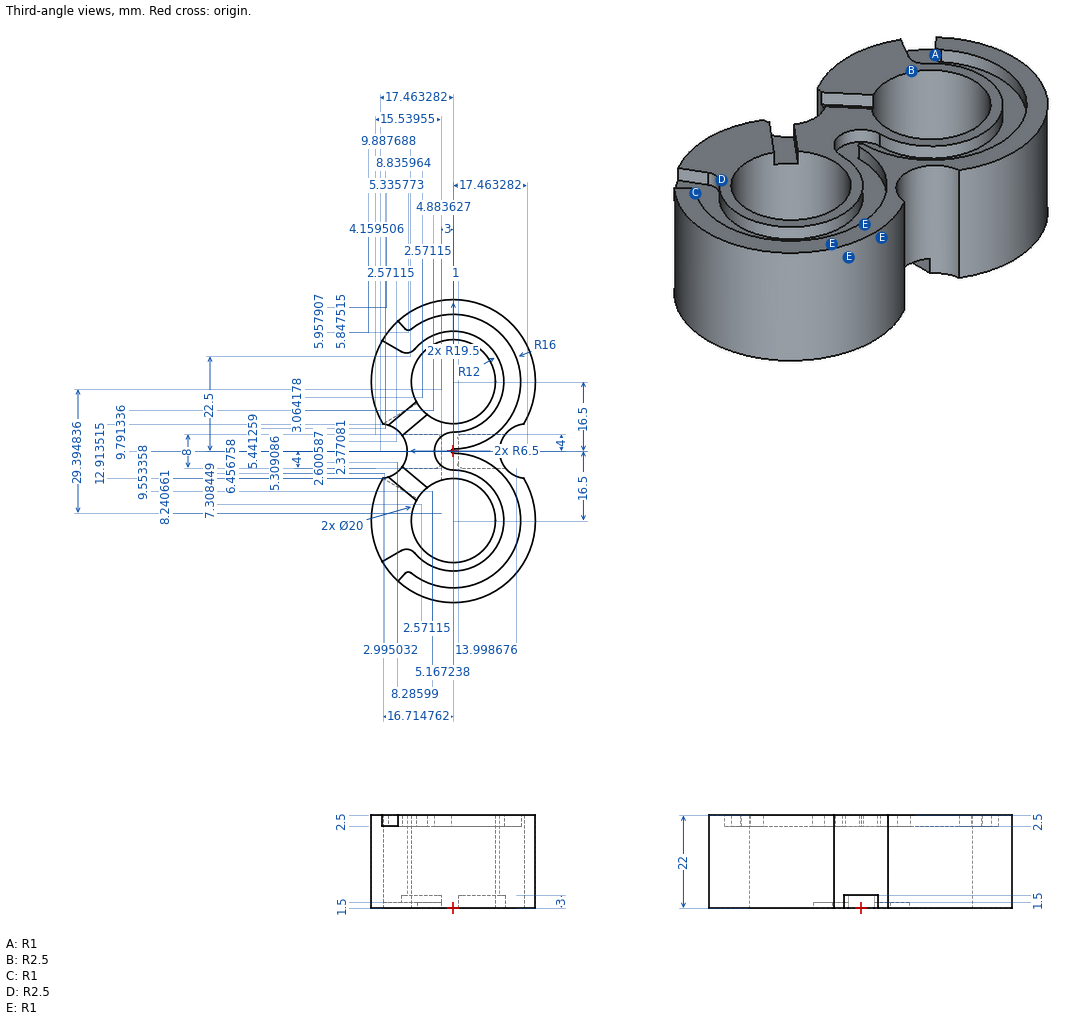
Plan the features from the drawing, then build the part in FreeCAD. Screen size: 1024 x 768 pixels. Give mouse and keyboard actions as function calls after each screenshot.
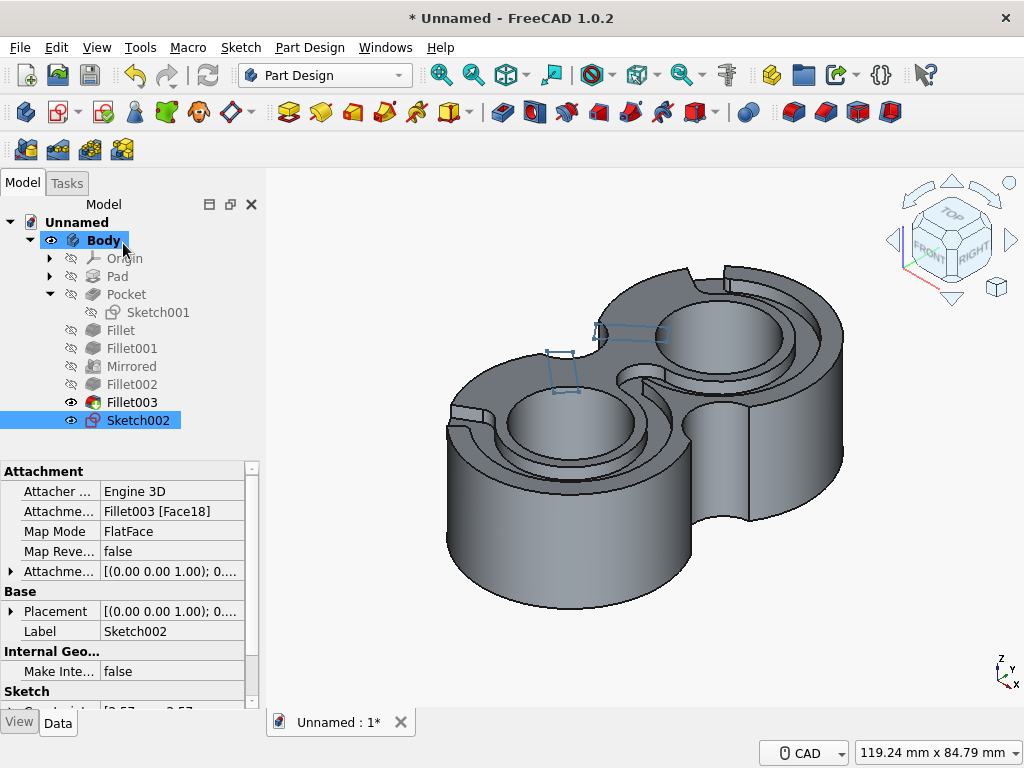
click(504, 112)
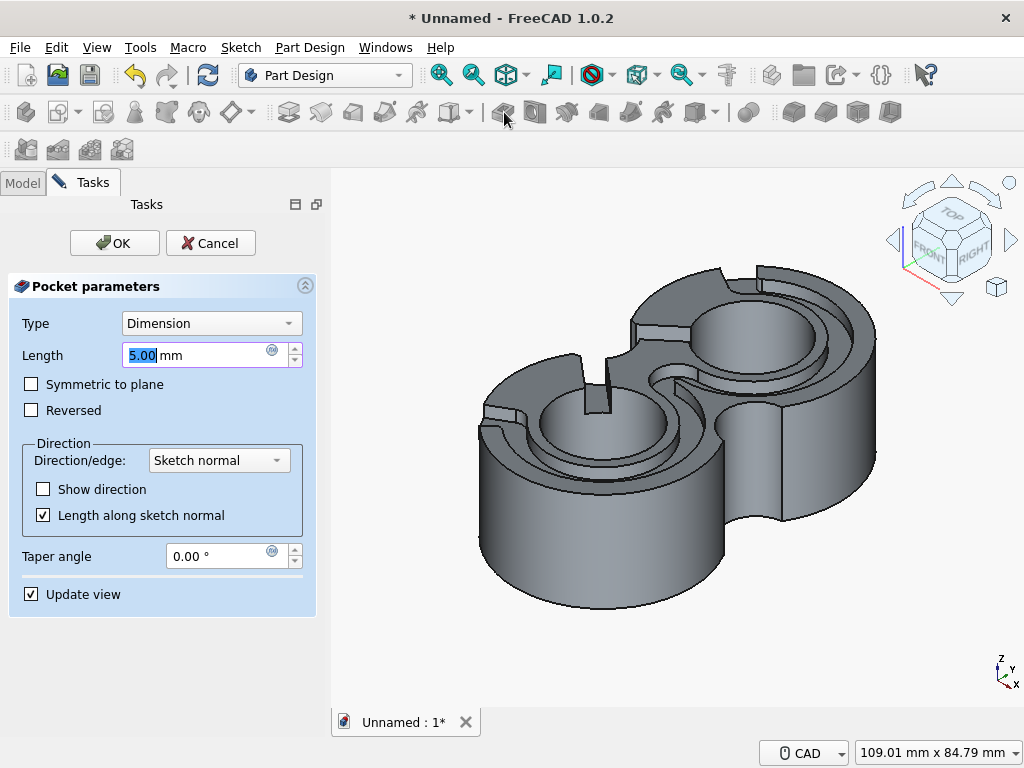
text(2.5)
key(Tab)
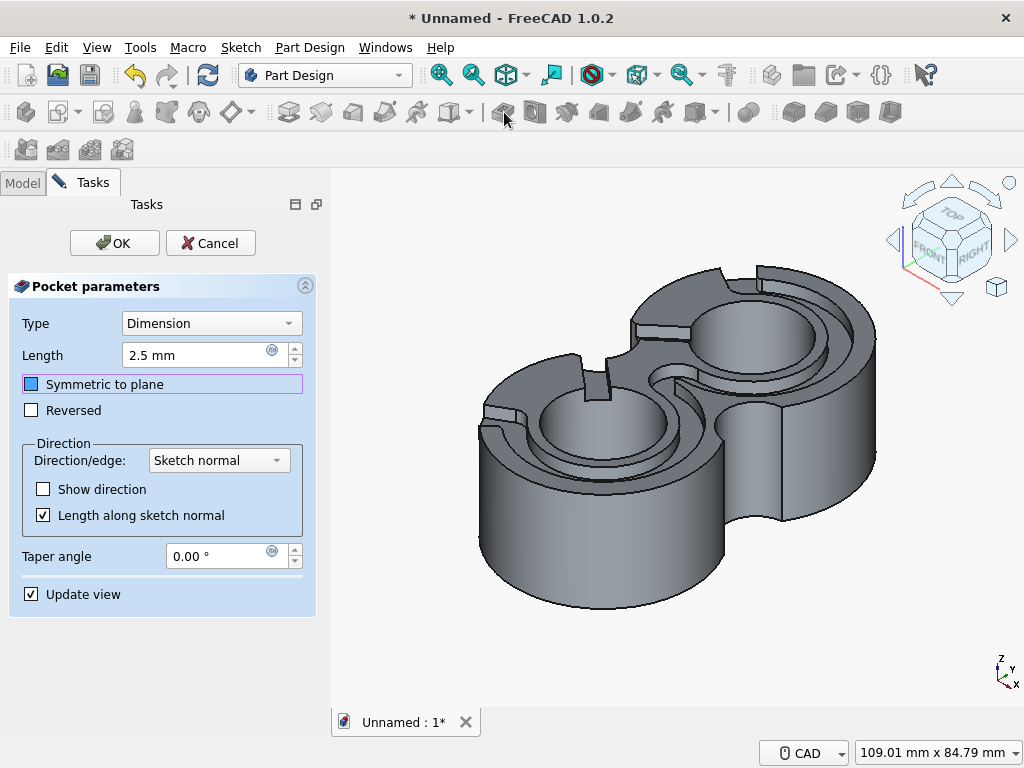
click(115, 243)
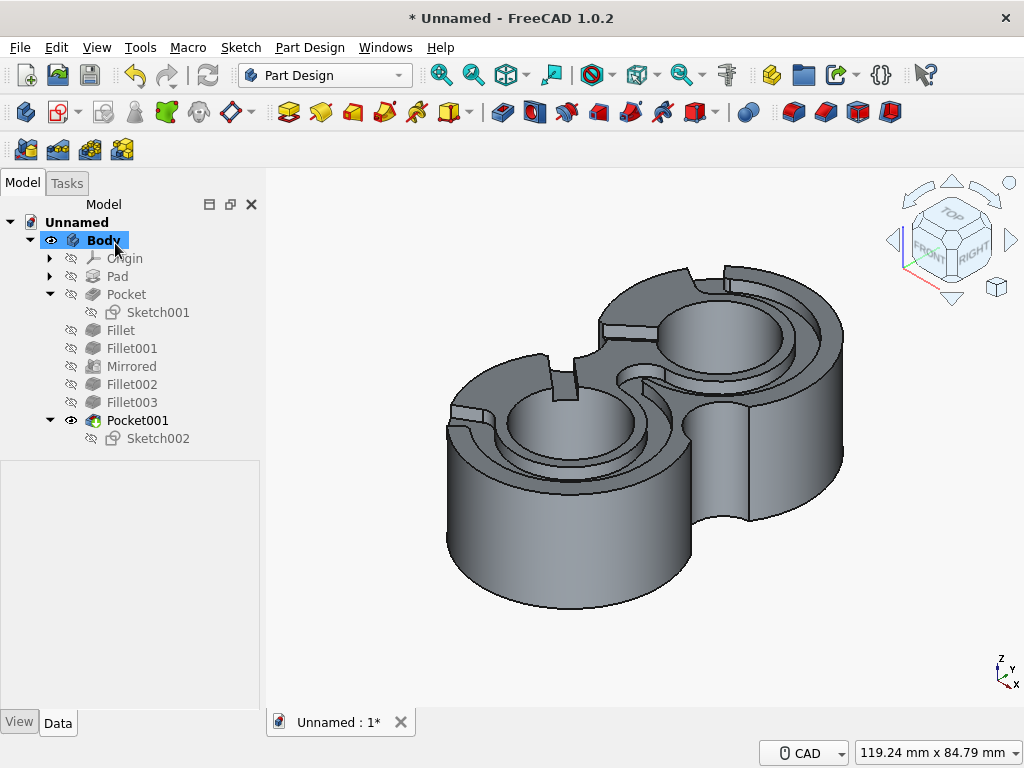
click(58, 112)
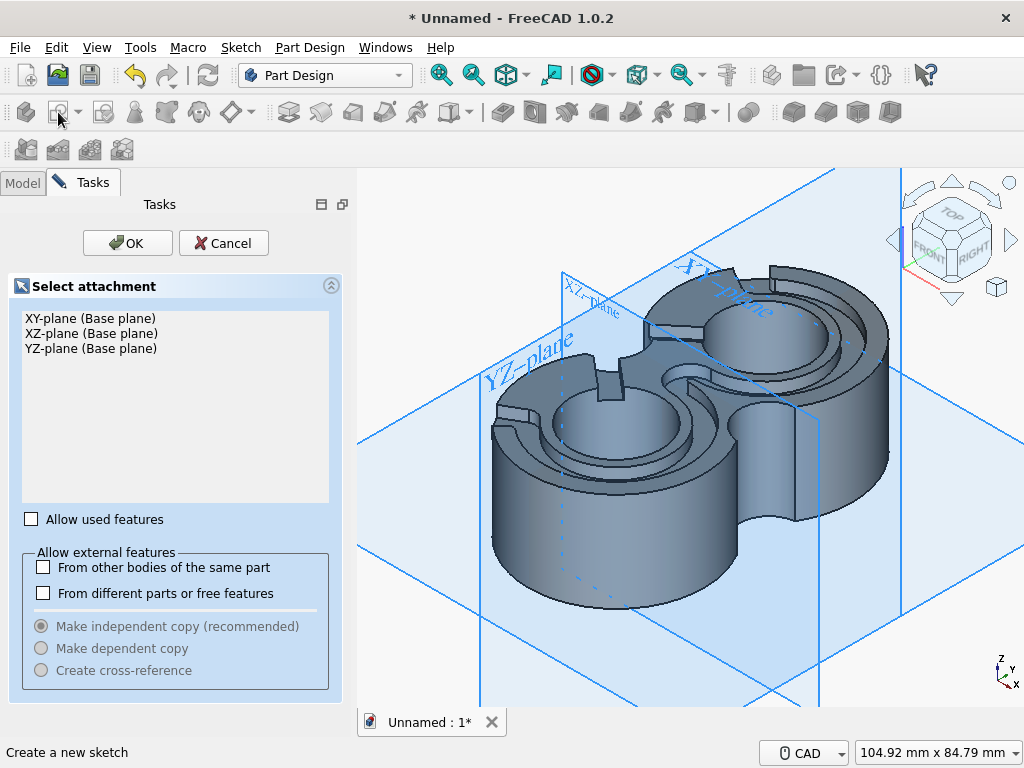
click(82, 318)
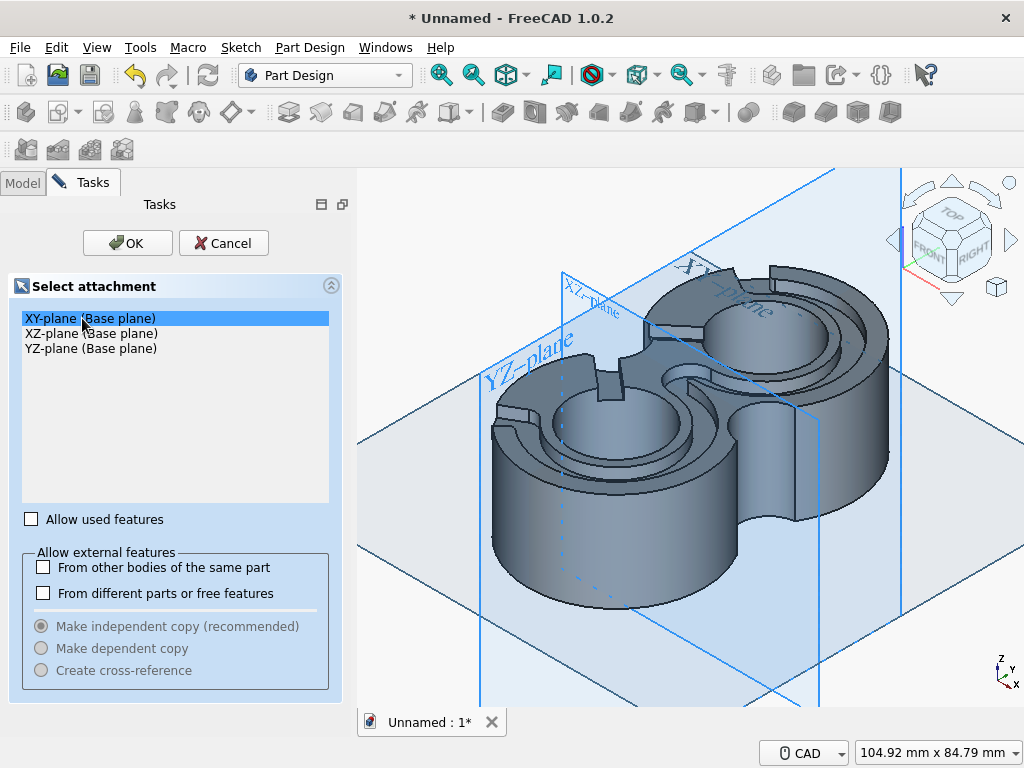
click(128, 243)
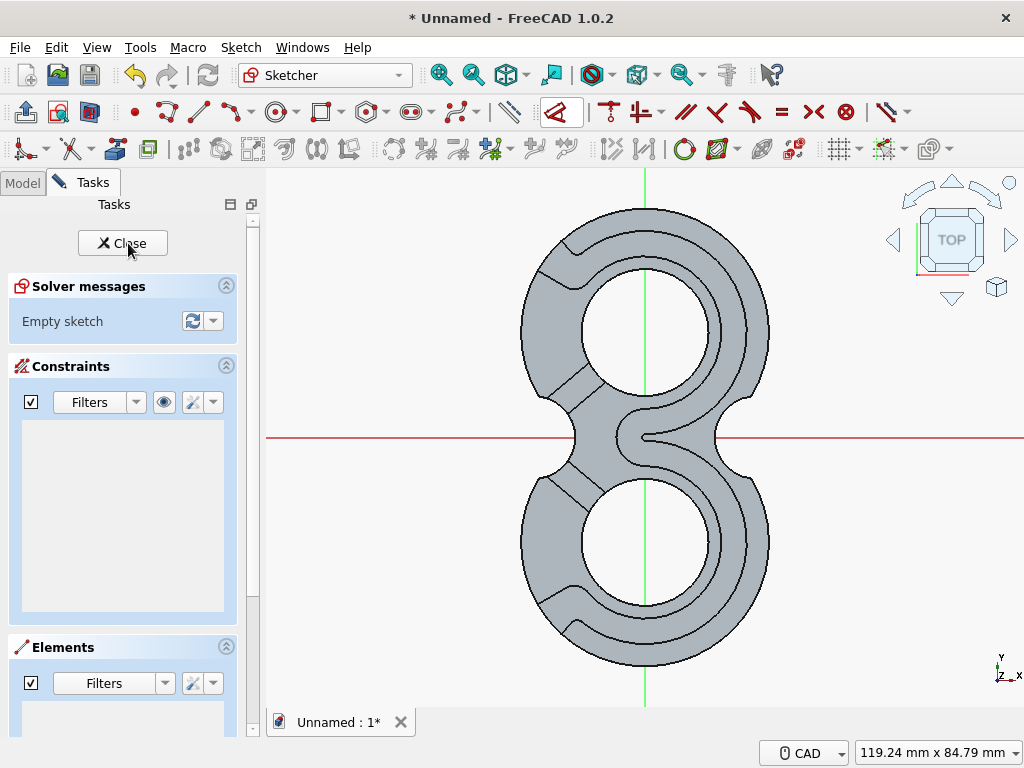
key(q)
key(s)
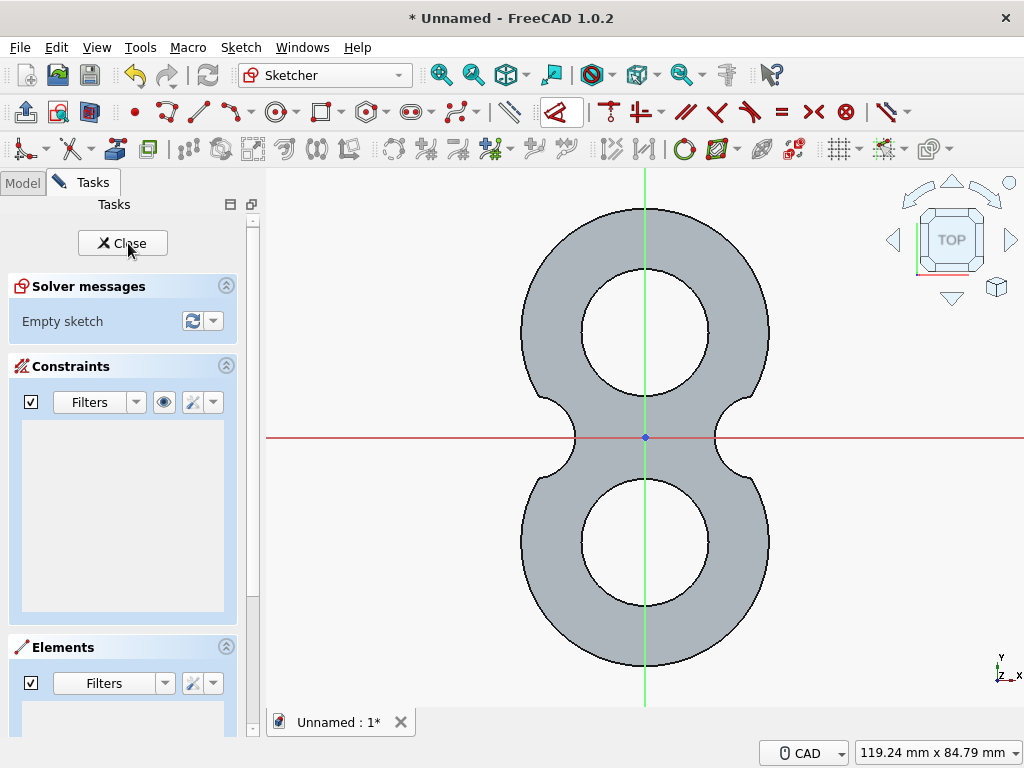
scroll(611, 437, up, 3)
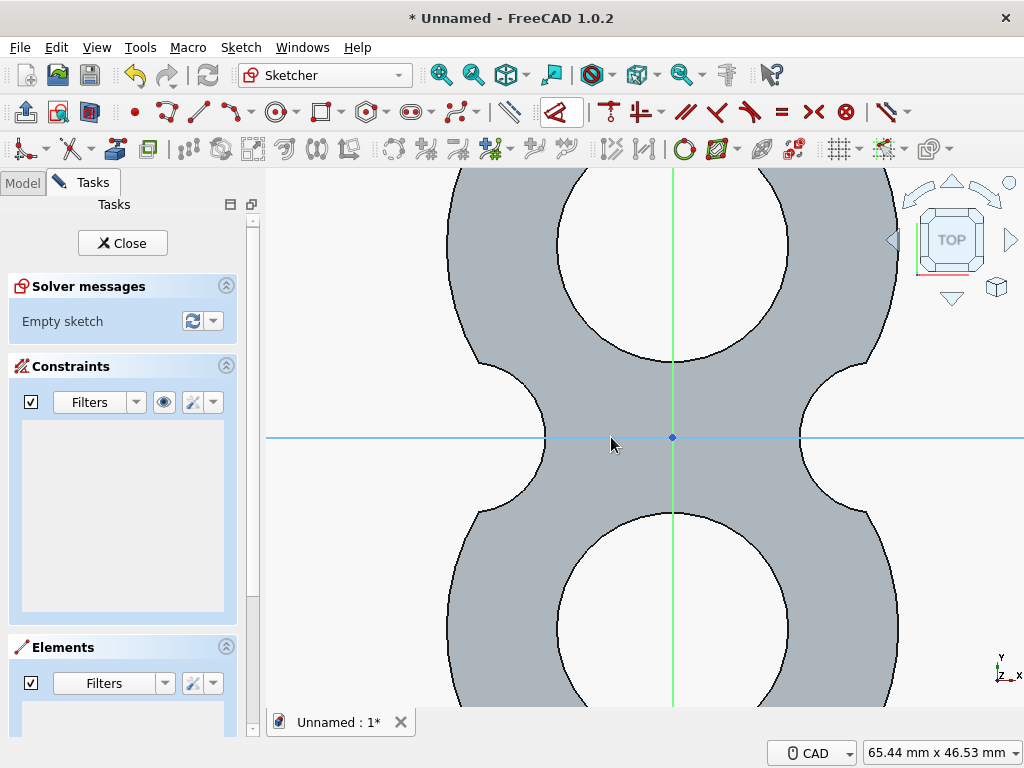
click(168, 112)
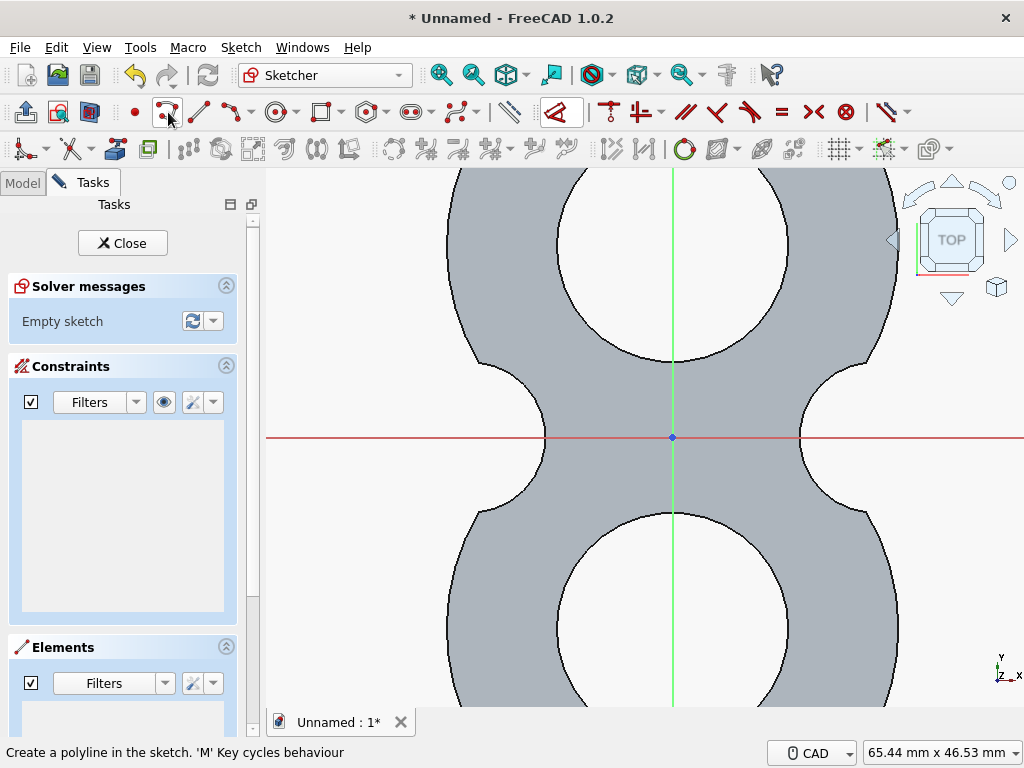
click(638, 267)
click(638, 608)
click(479, 512)
click(479, 363)
click(638, 268)
key(Escape)
key(Escape)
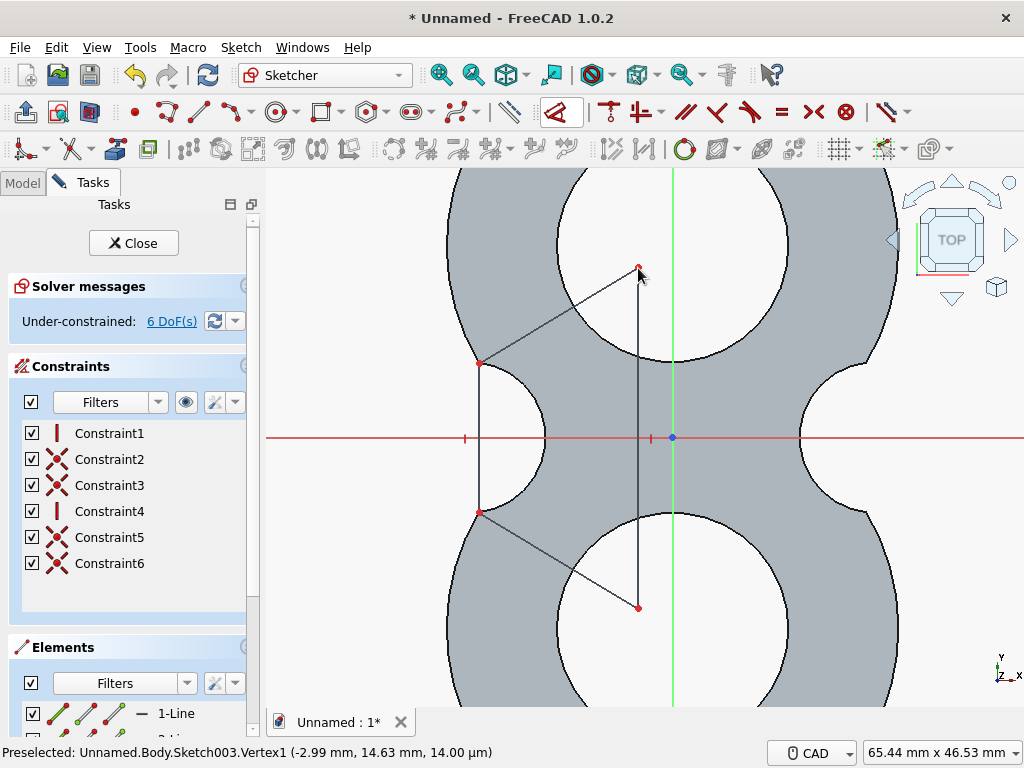
click(638, 268)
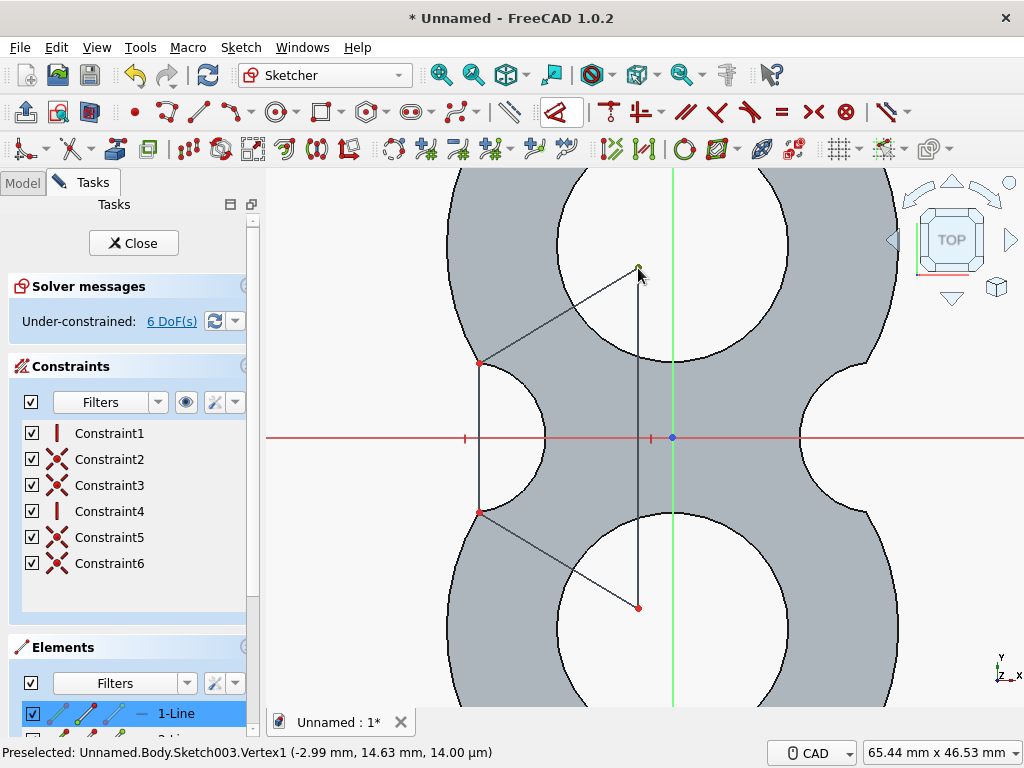
key(l)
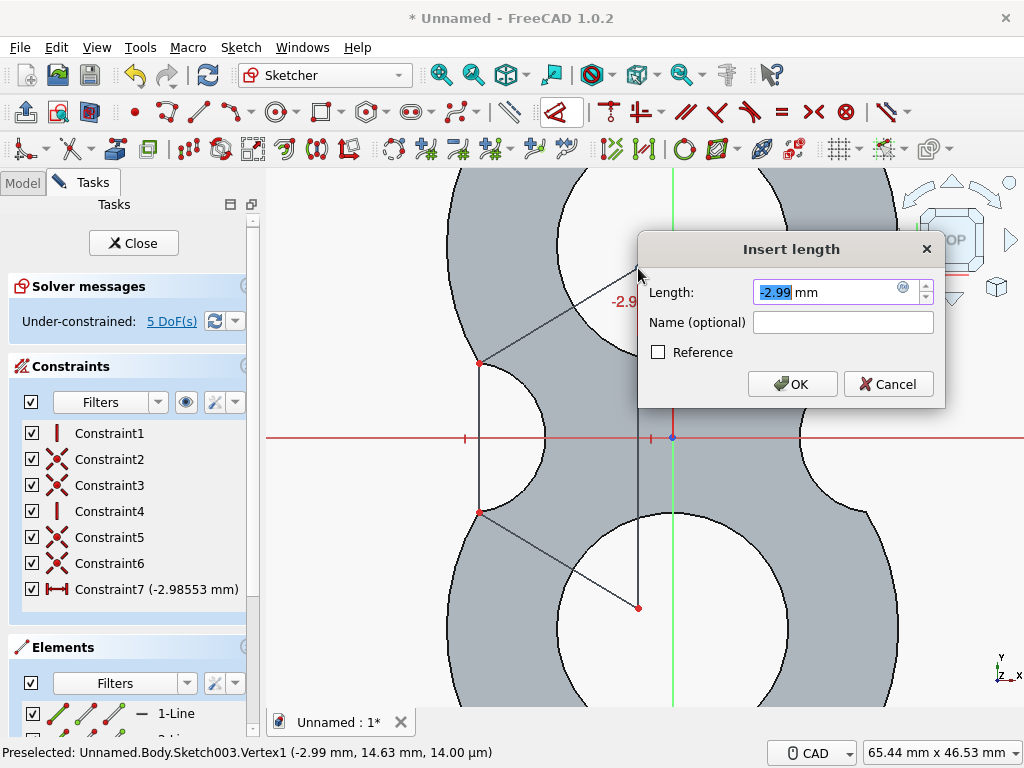
text(-3)
key(Return)